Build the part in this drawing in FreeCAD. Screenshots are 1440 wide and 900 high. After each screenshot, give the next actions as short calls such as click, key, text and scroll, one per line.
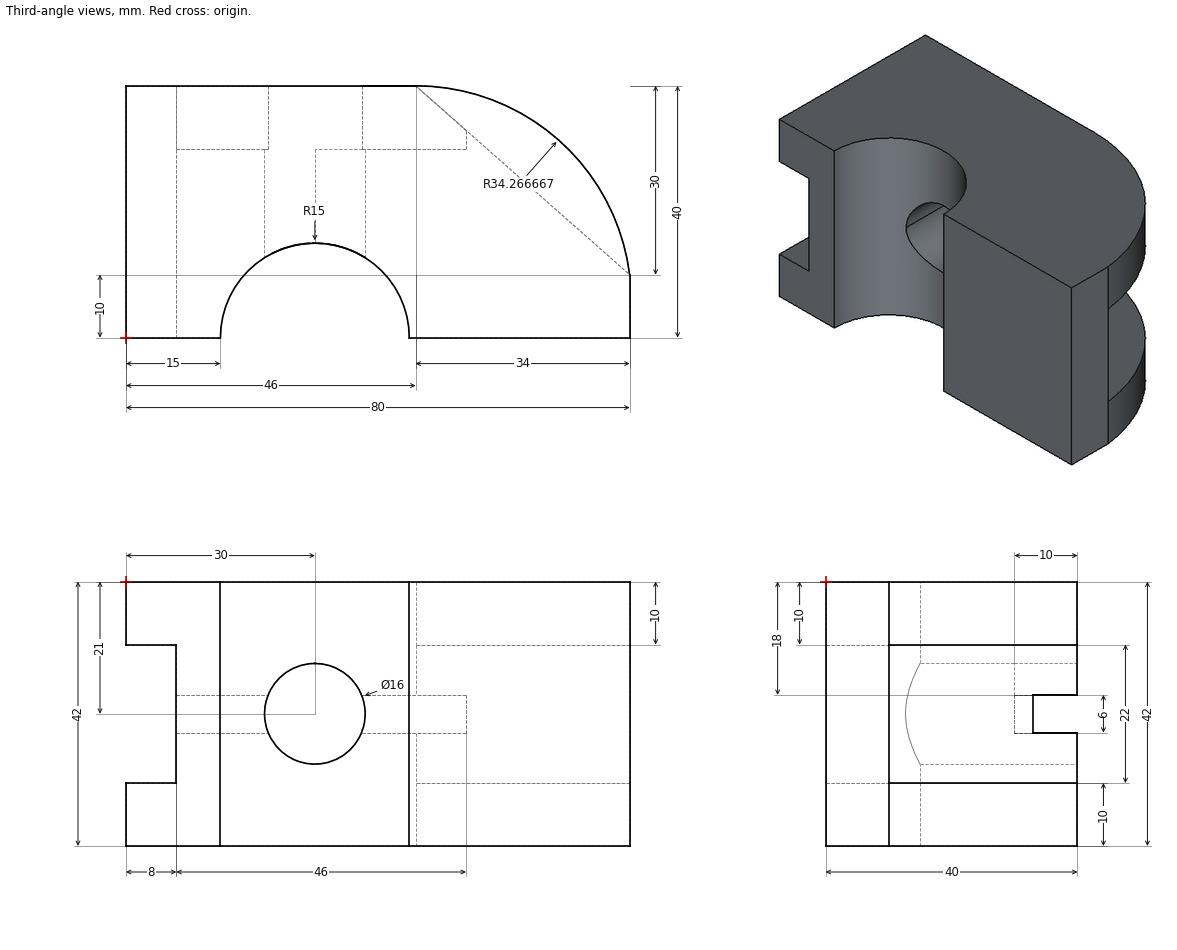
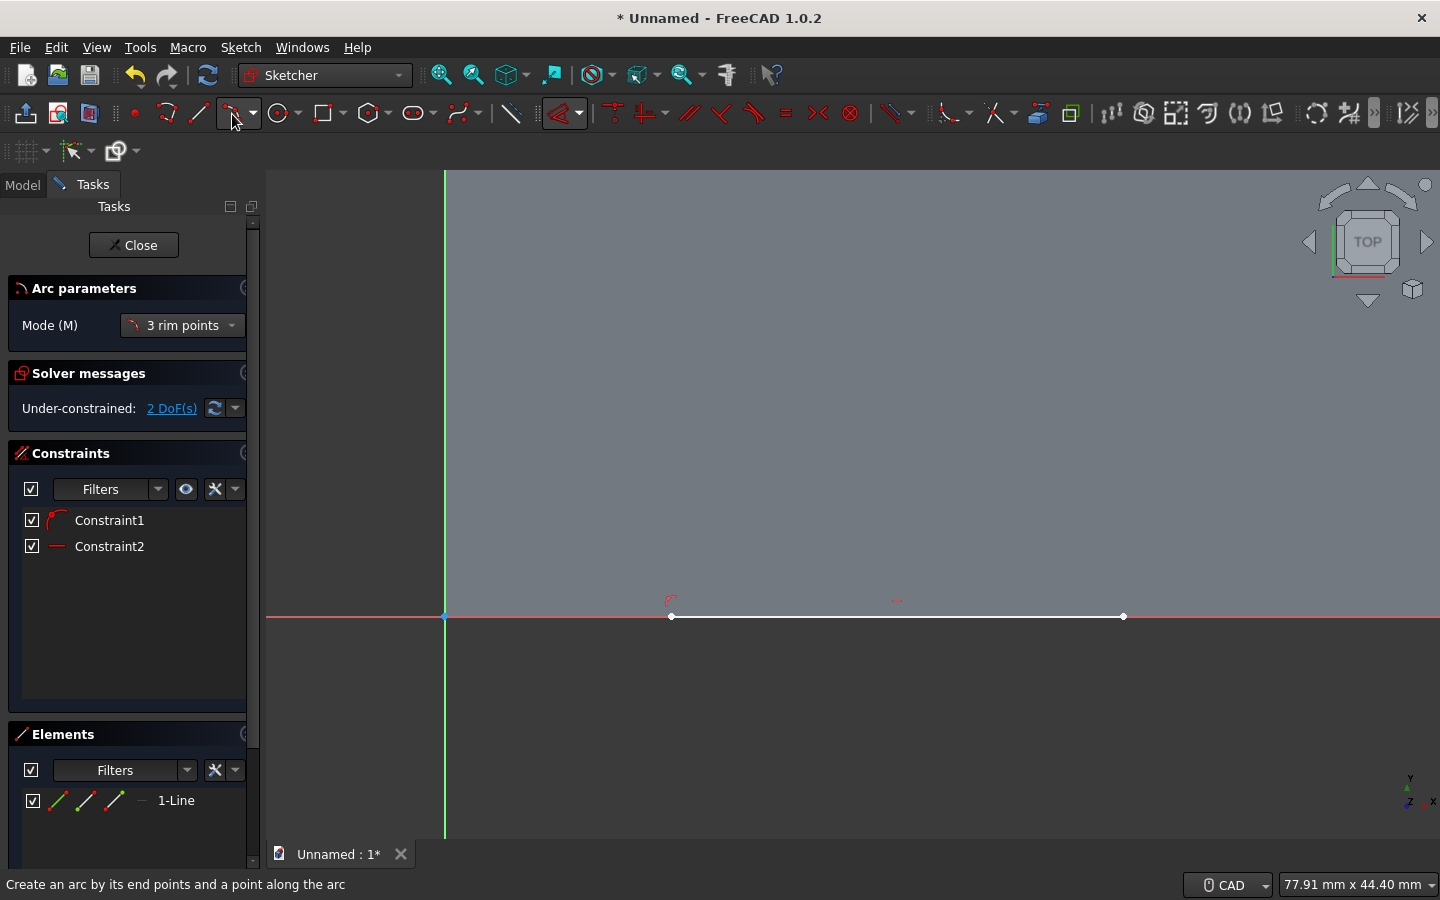
click(1123, 617)
click(671, 617)
click(897, 391)
key(Escape)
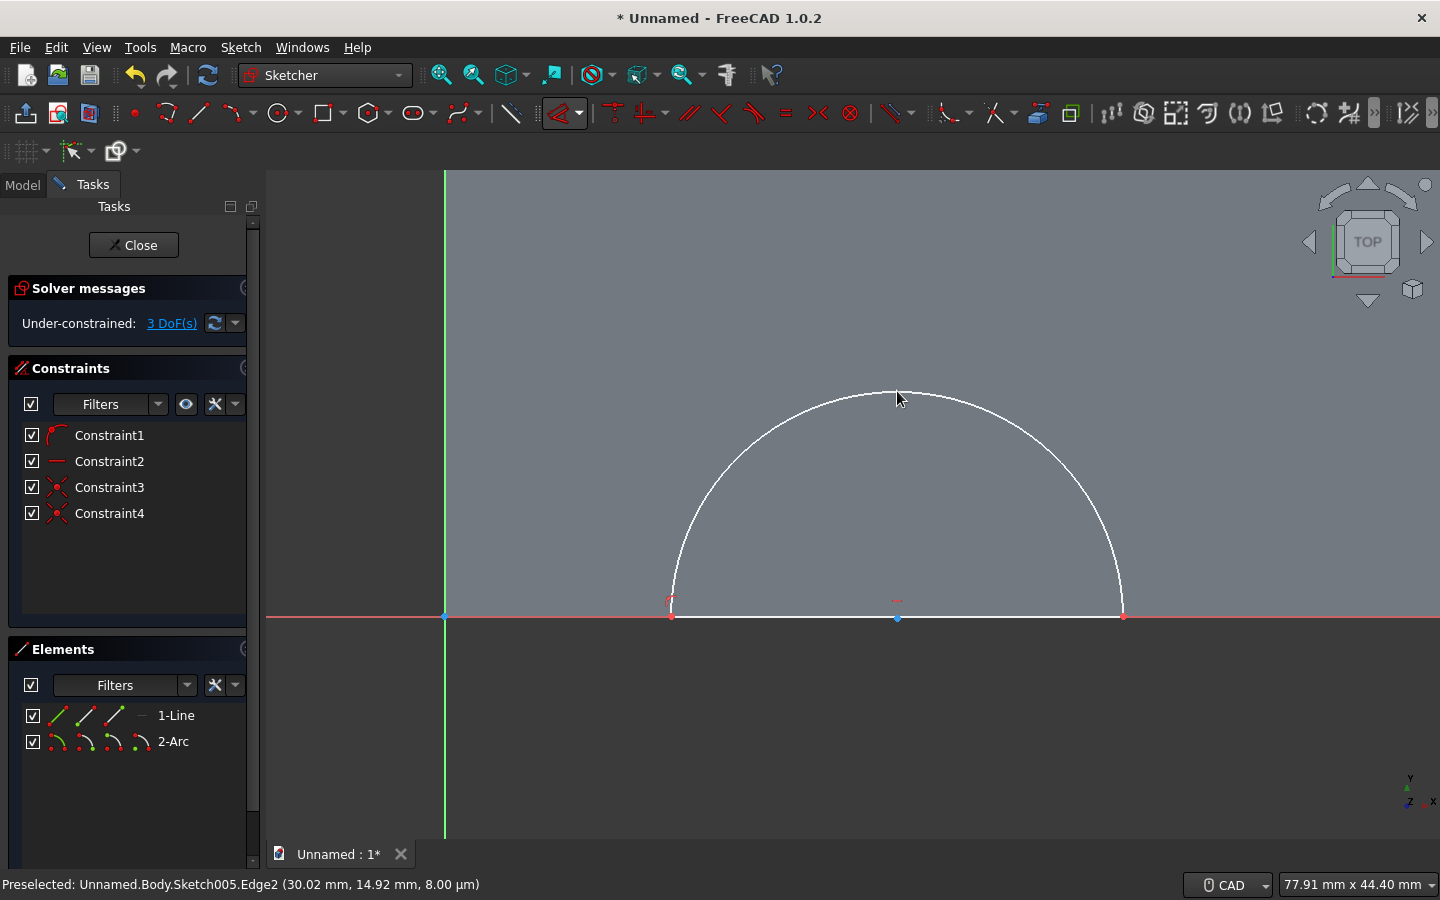
click(897, 618)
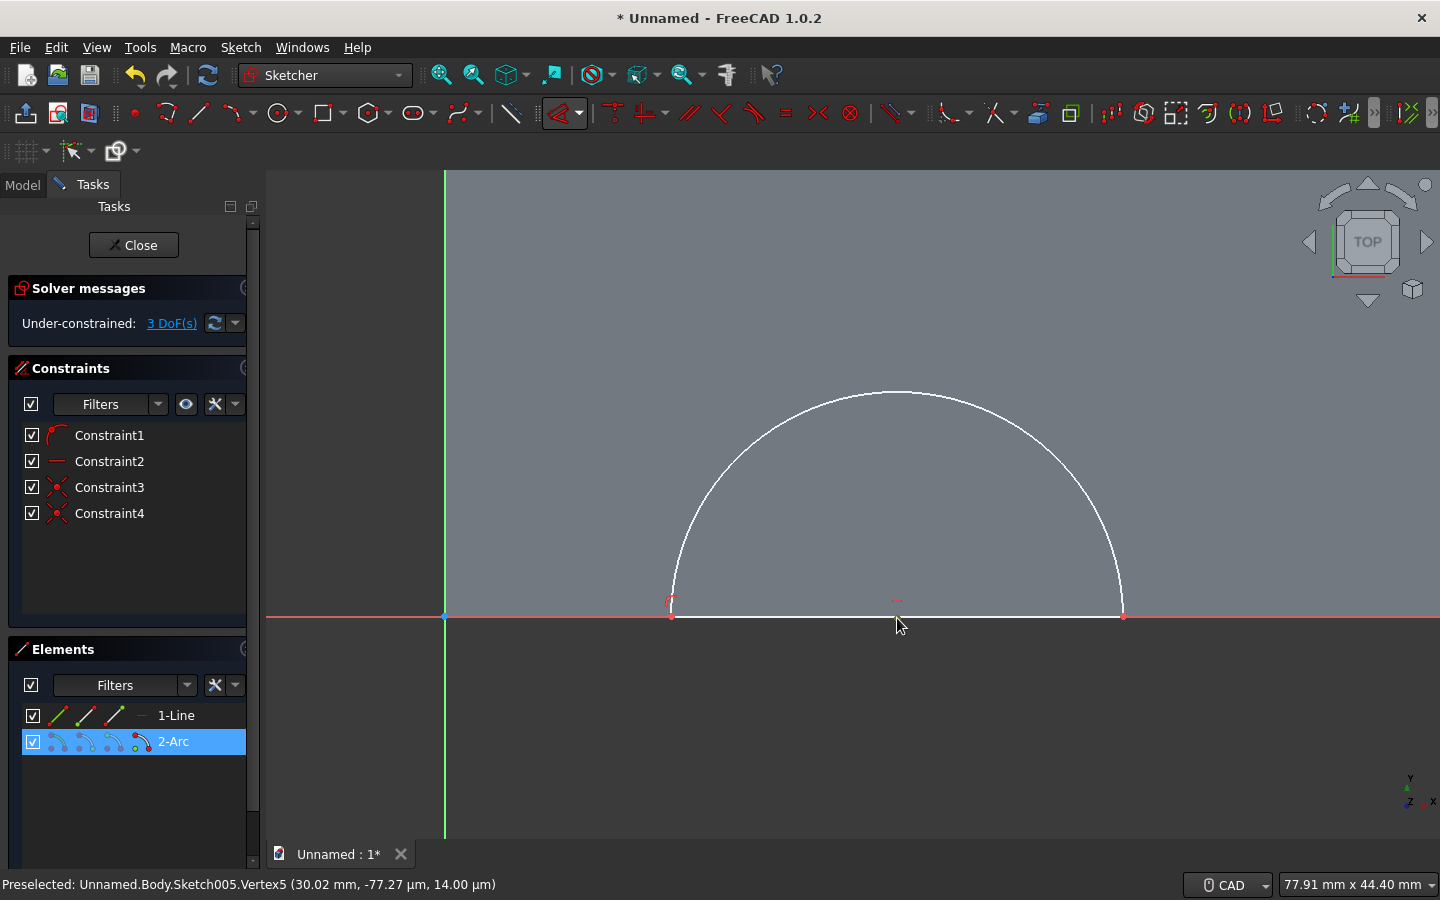
click(364, 617)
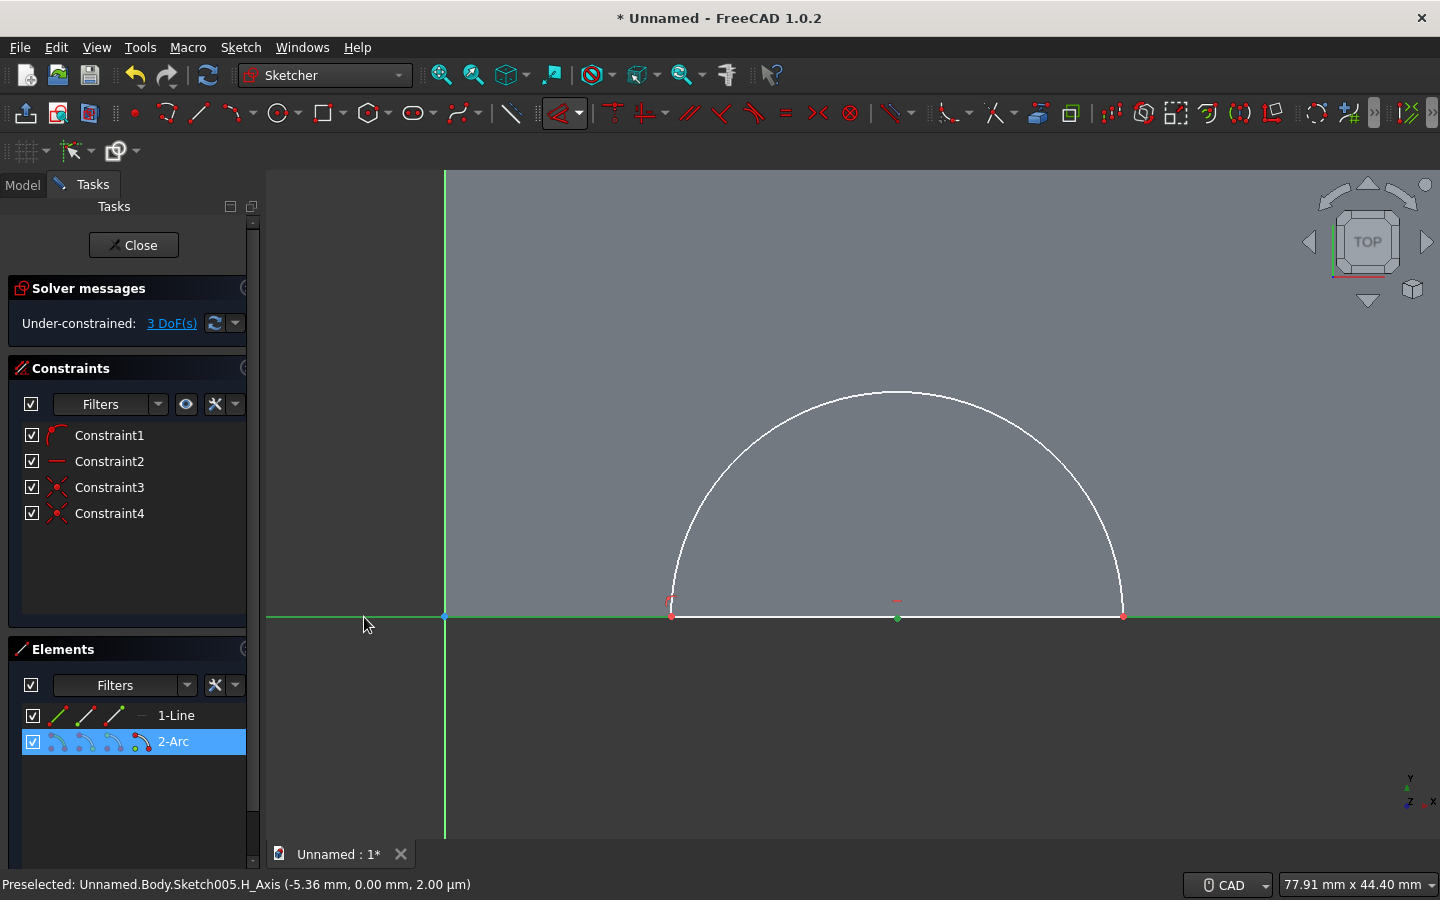
click(614, 114)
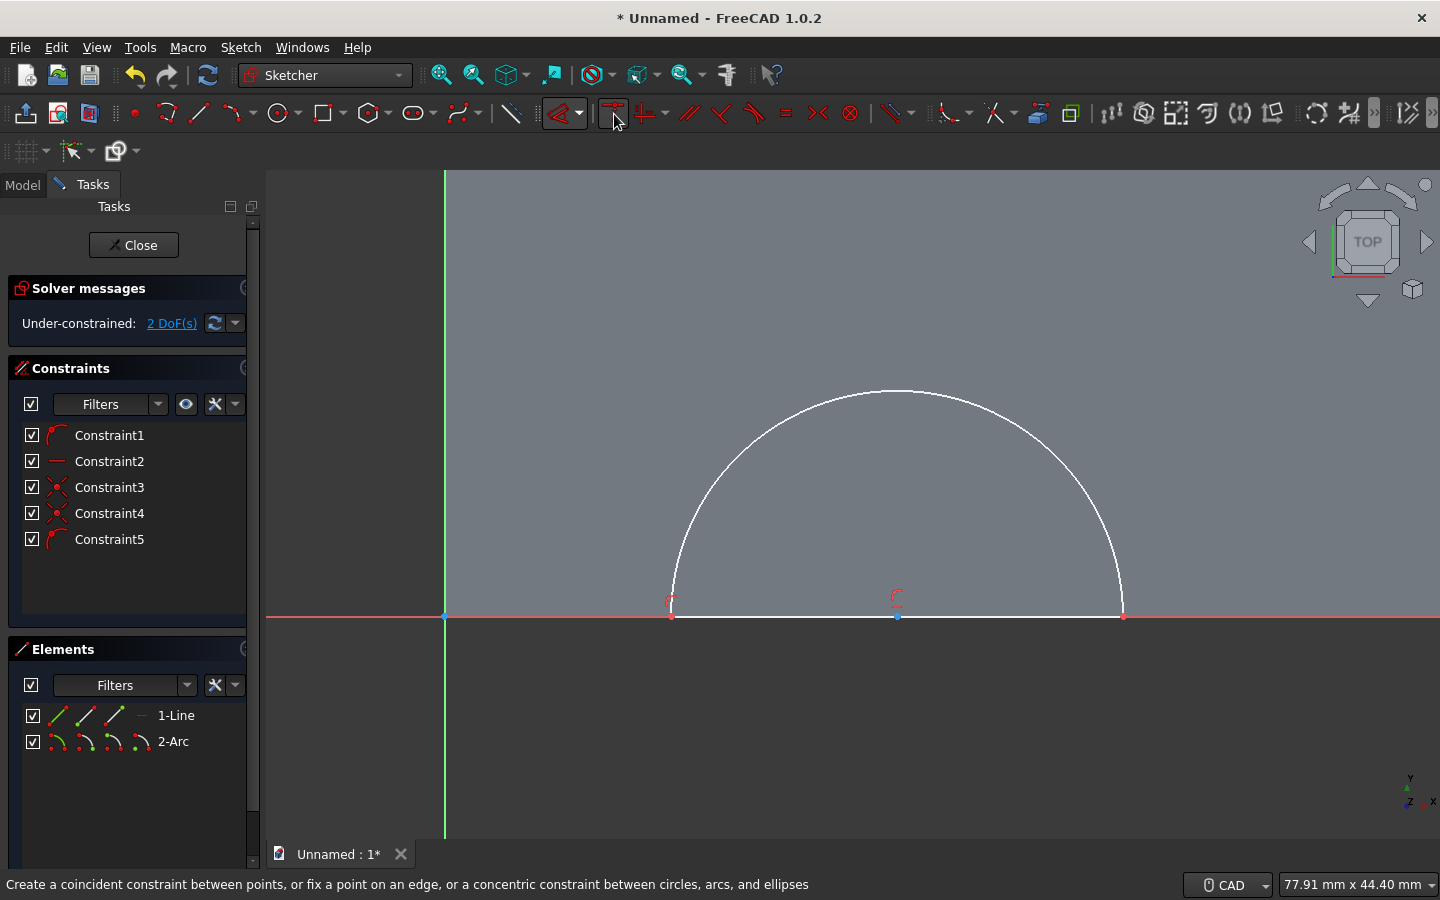
click(1030, 434)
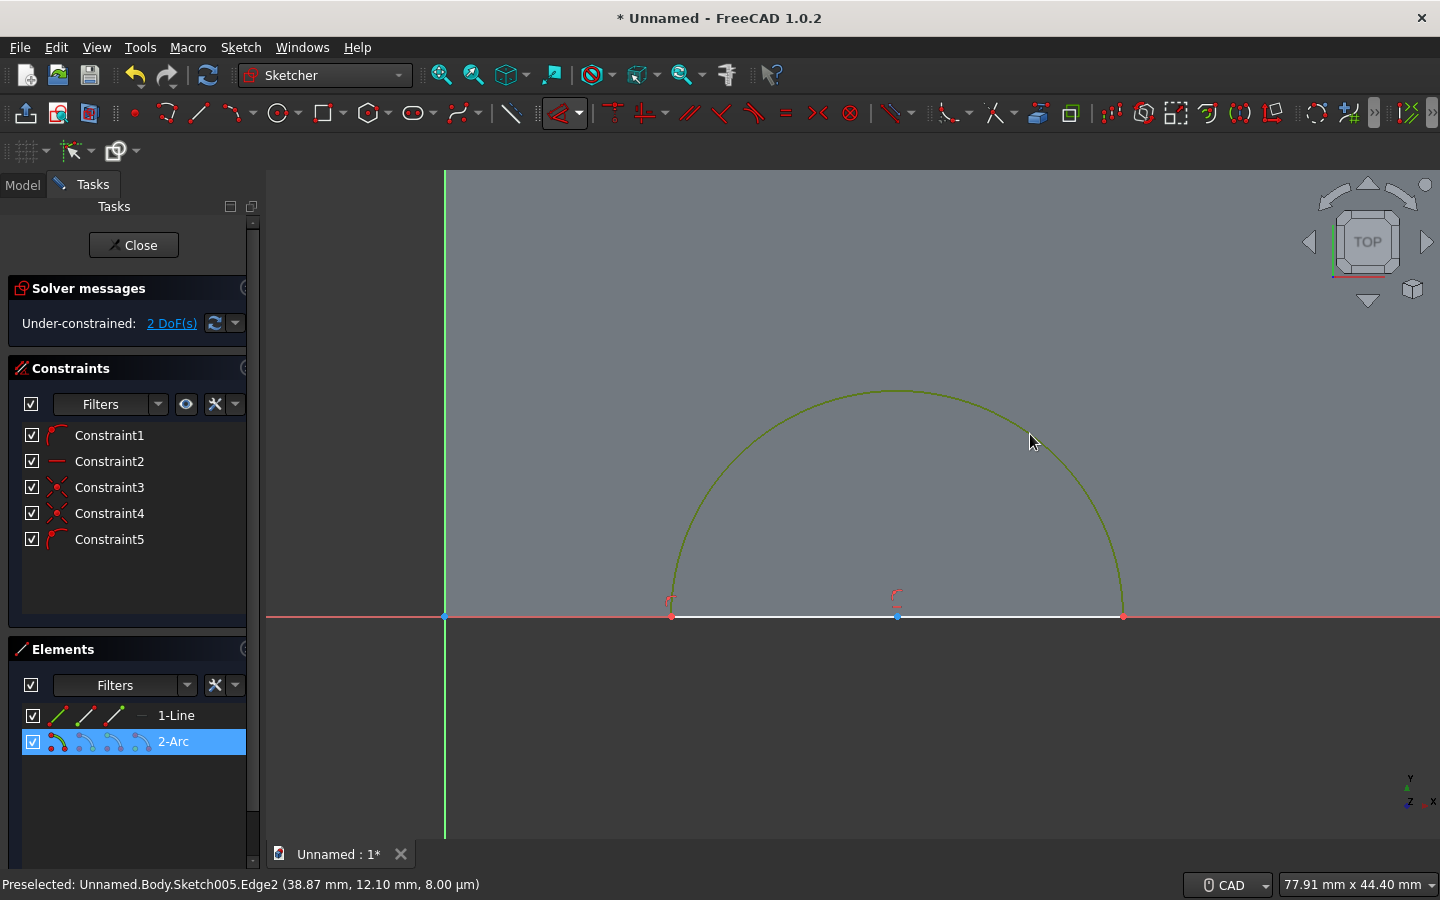
key(k)
key(r)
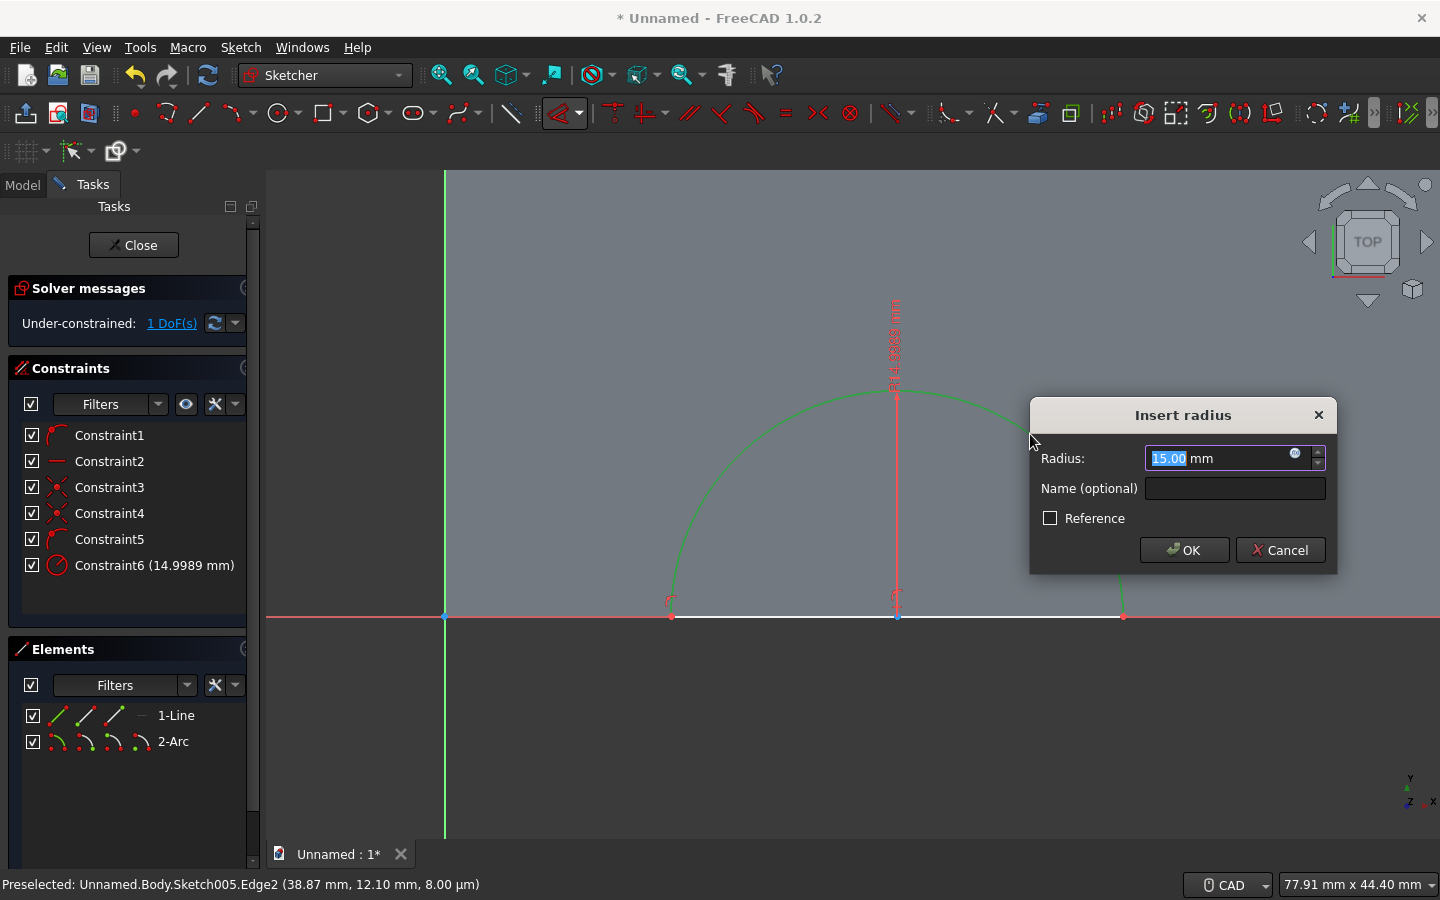
text(15)
key(Return)